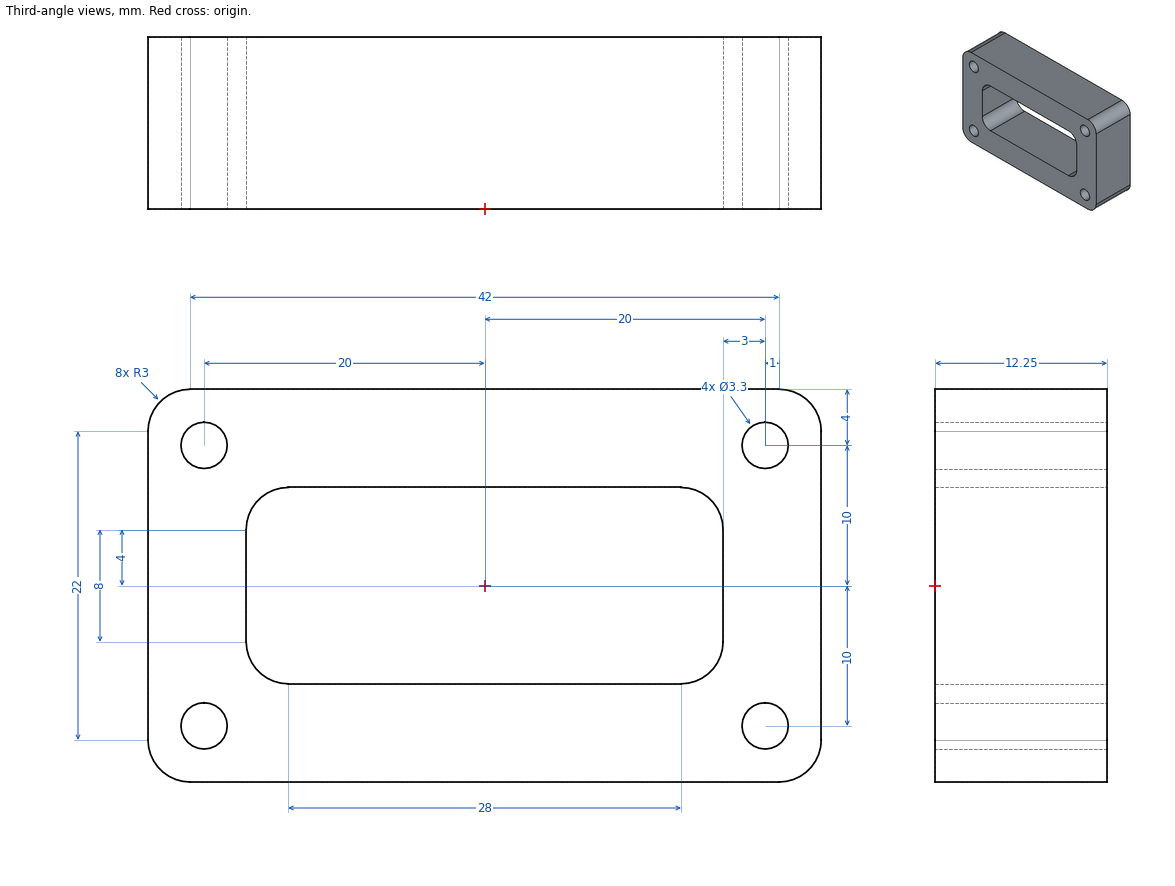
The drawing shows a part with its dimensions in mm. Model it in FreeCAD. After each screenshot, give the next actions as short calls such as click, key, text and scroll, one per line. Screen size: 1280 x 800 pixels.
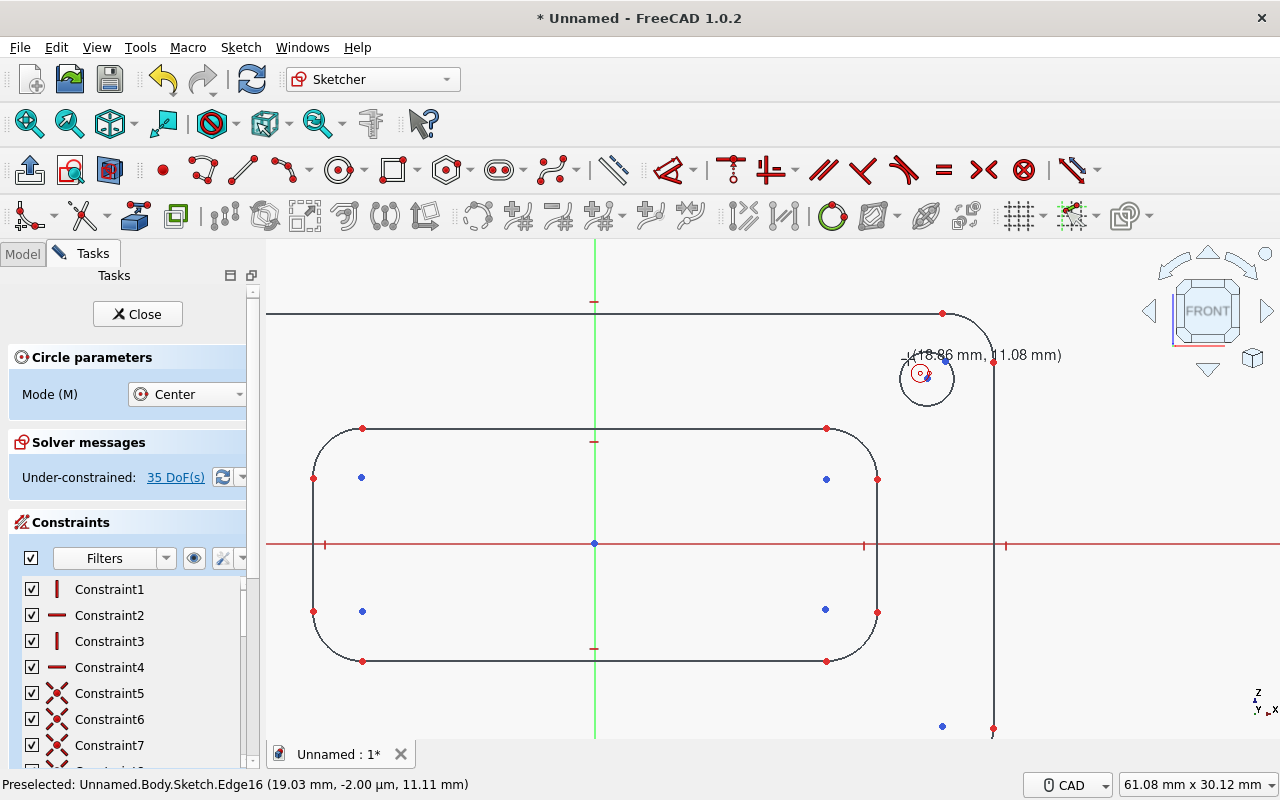
scroll(927, 377, down, 2)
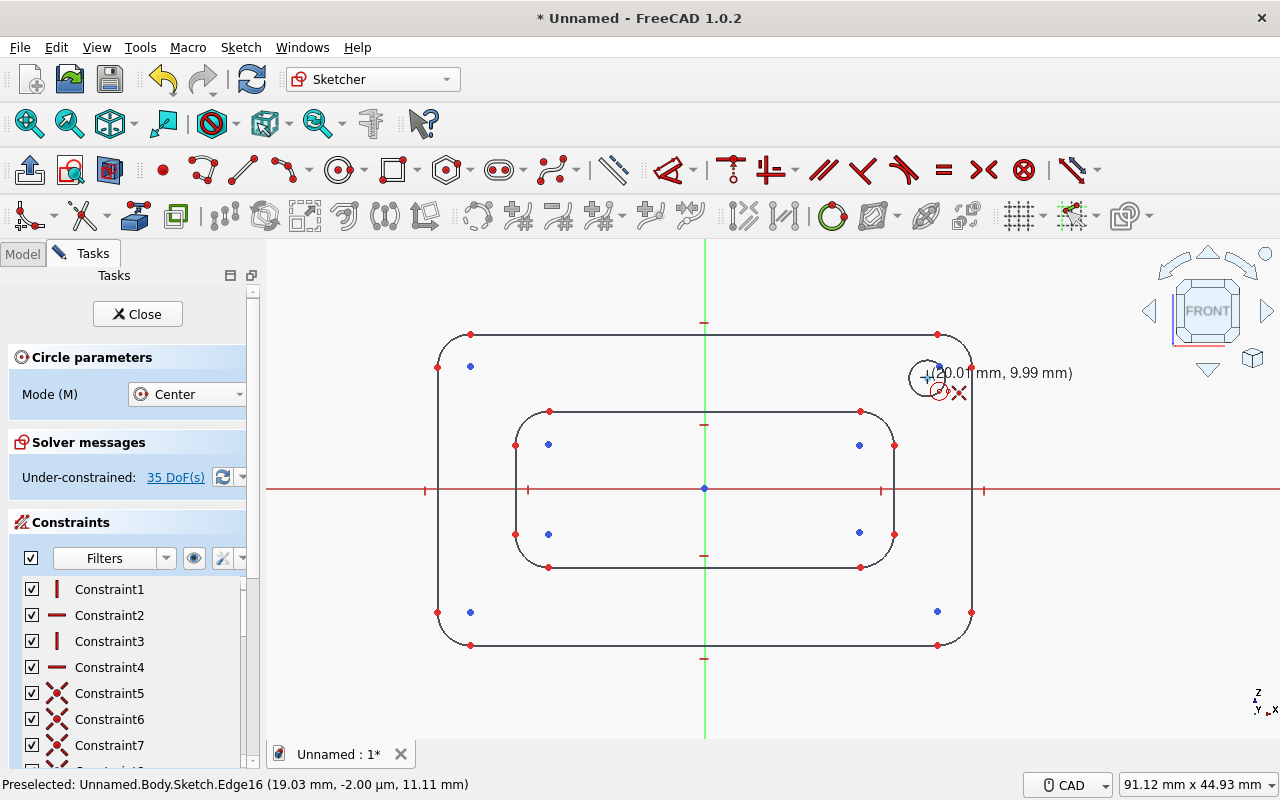
scroll(482, 378, up, 2)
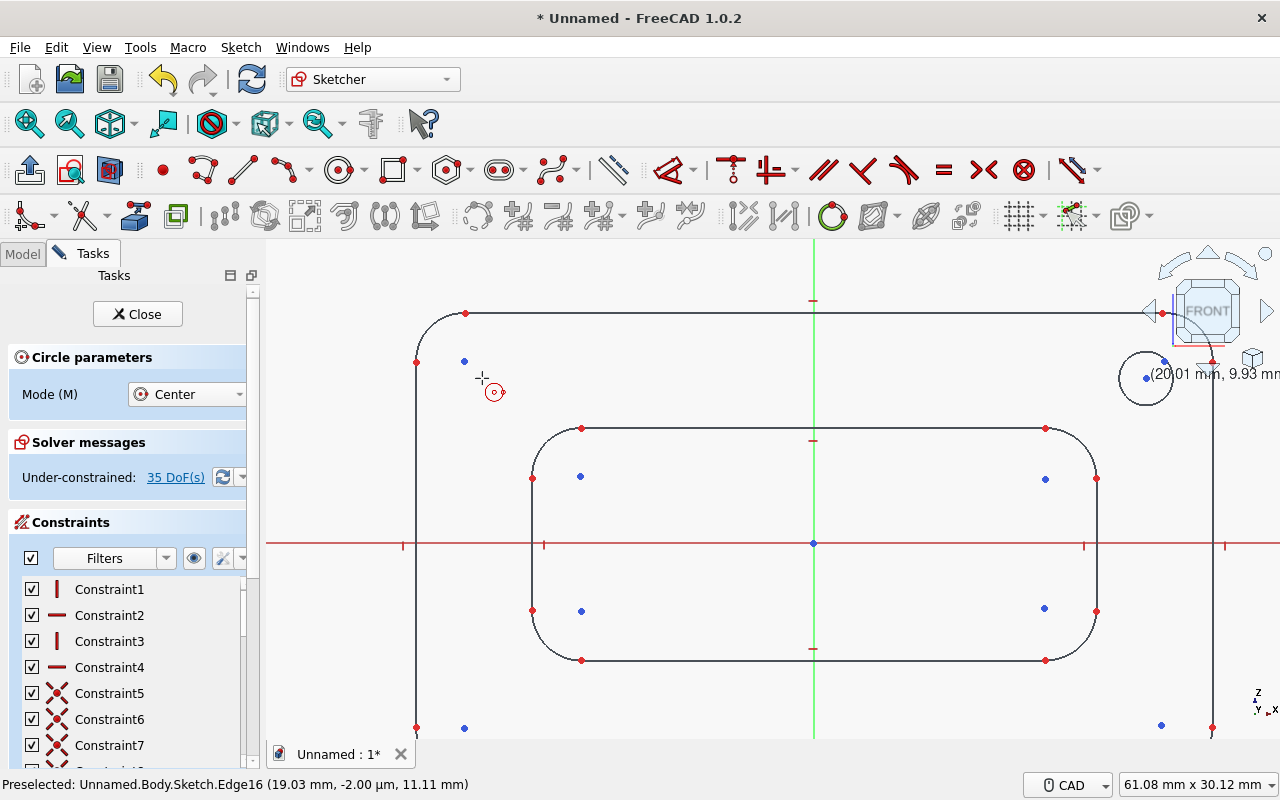
click(482, 377)
click(501, 358)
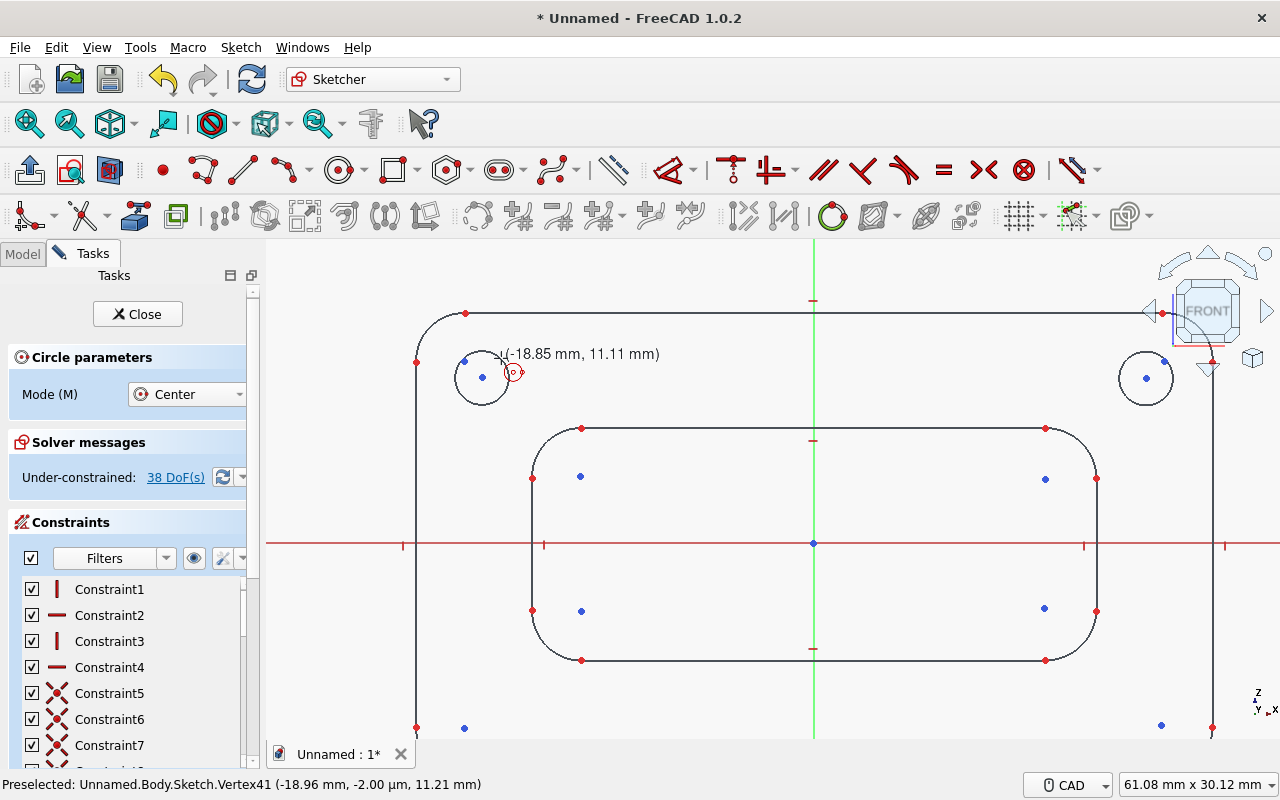
scroll(482, 378, down, 2)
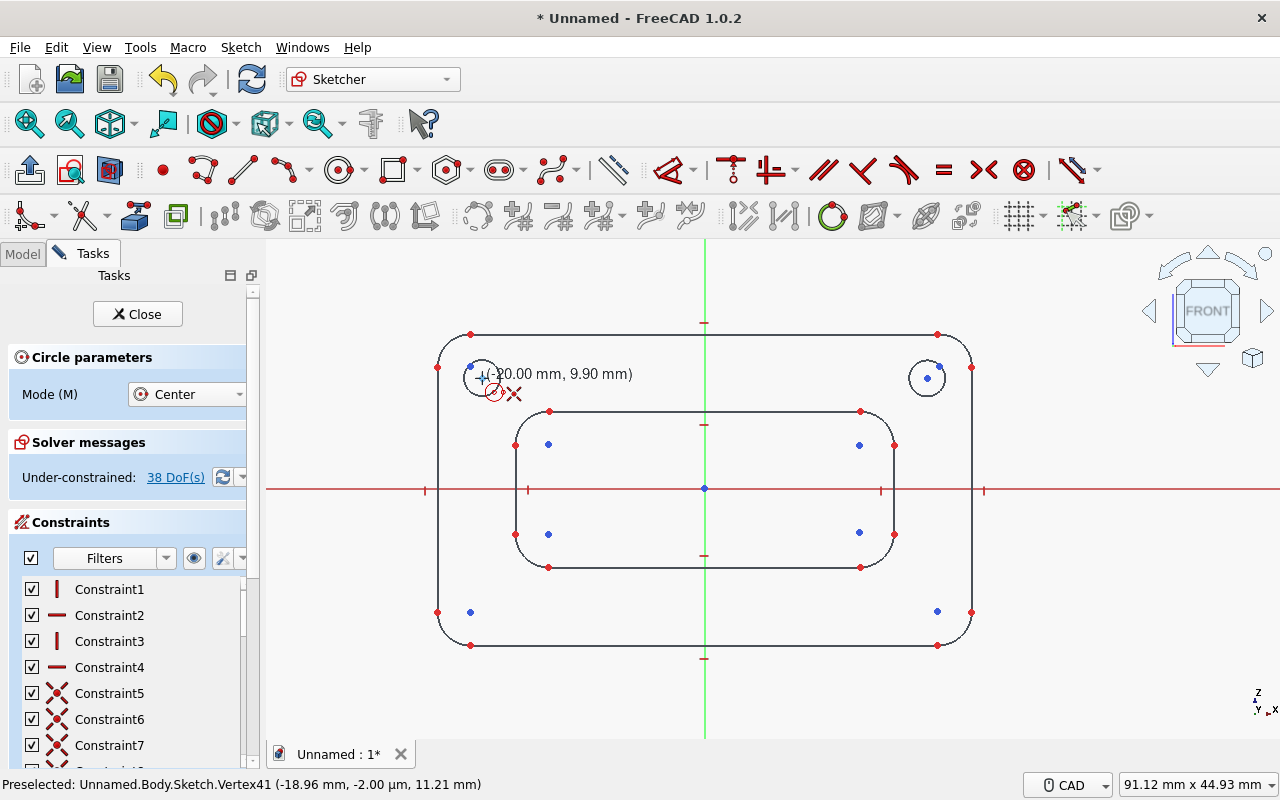
scroll(927, 600, up, 2)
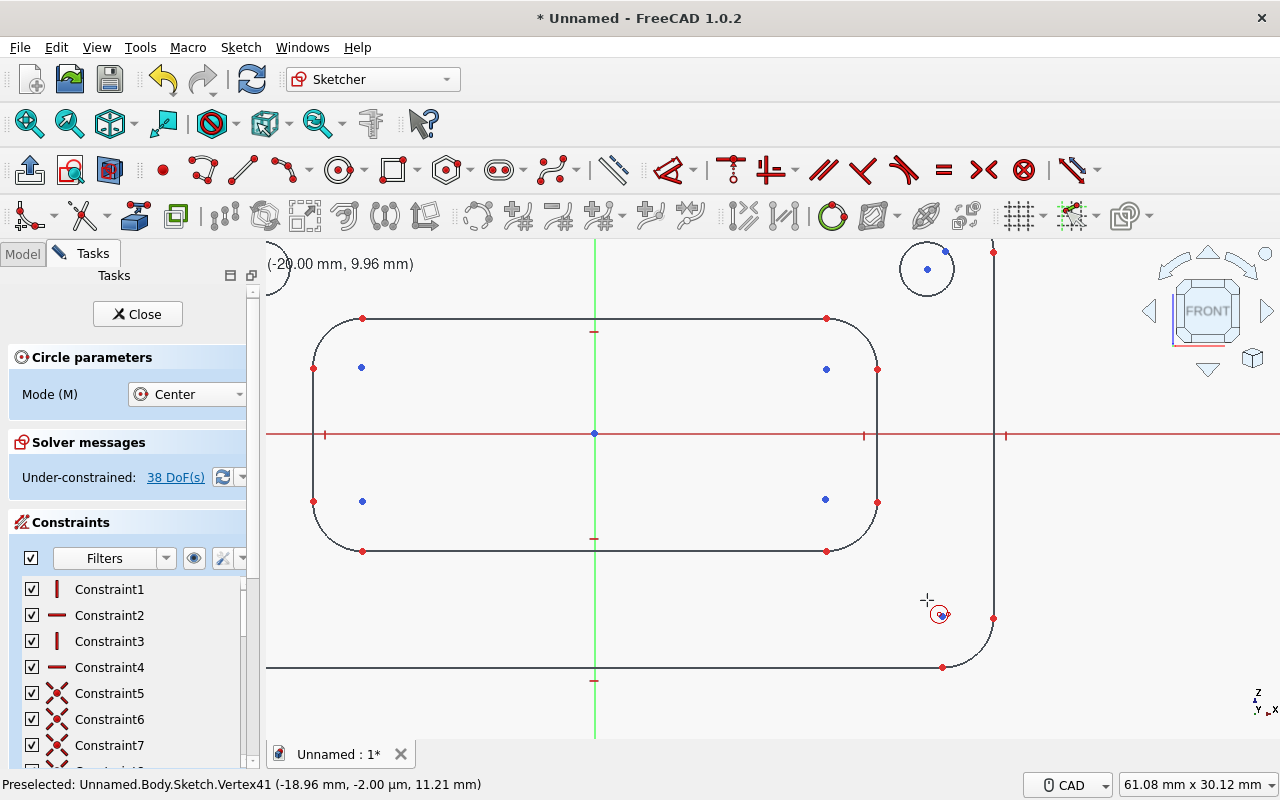
click(927, 600)
click(946, 581)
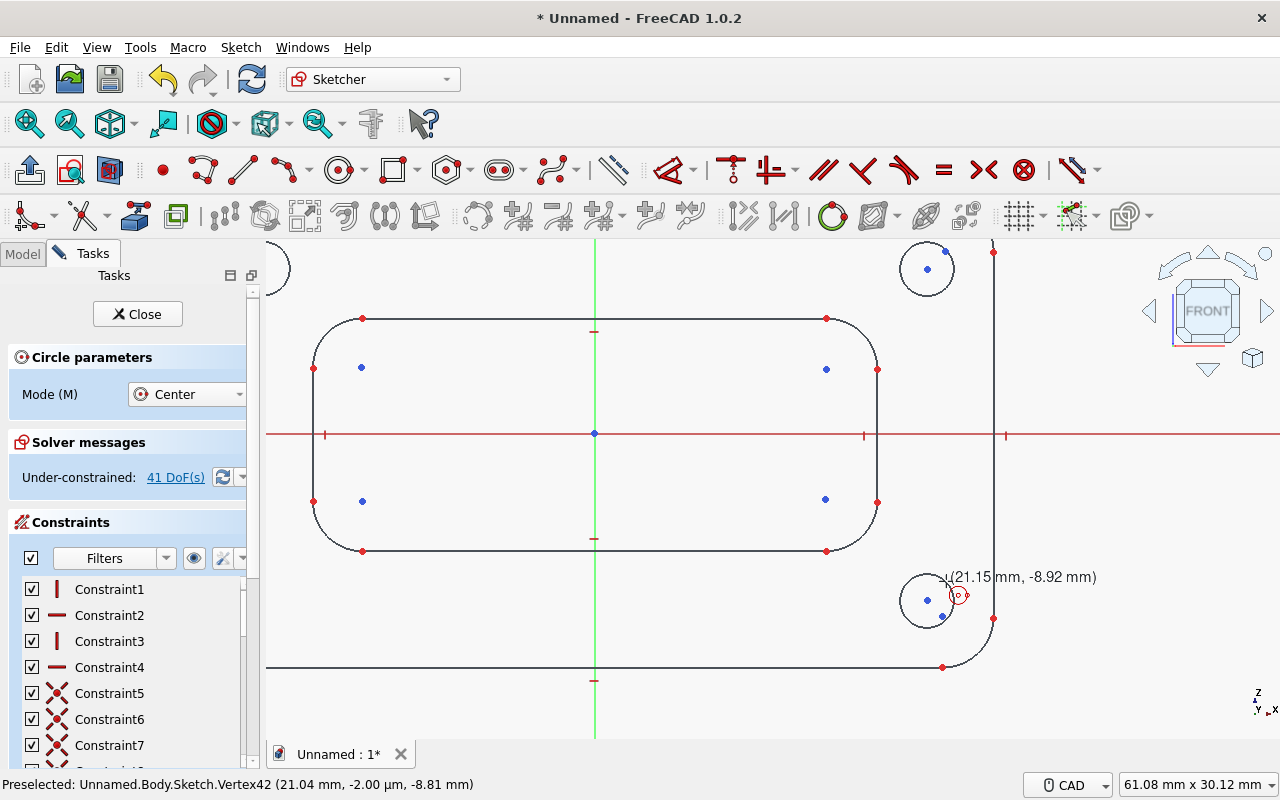
scroll(927, 601, down, 2)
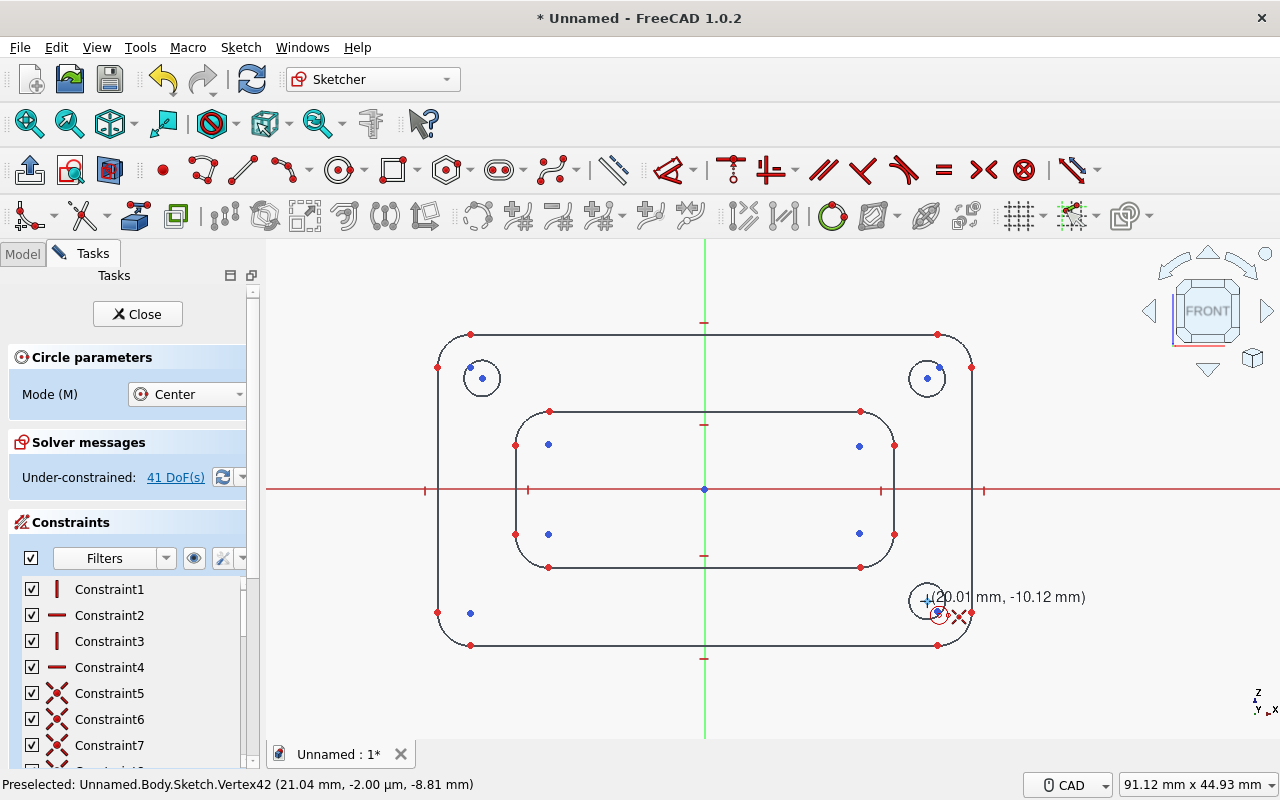
scroll(482, 601, up, 2)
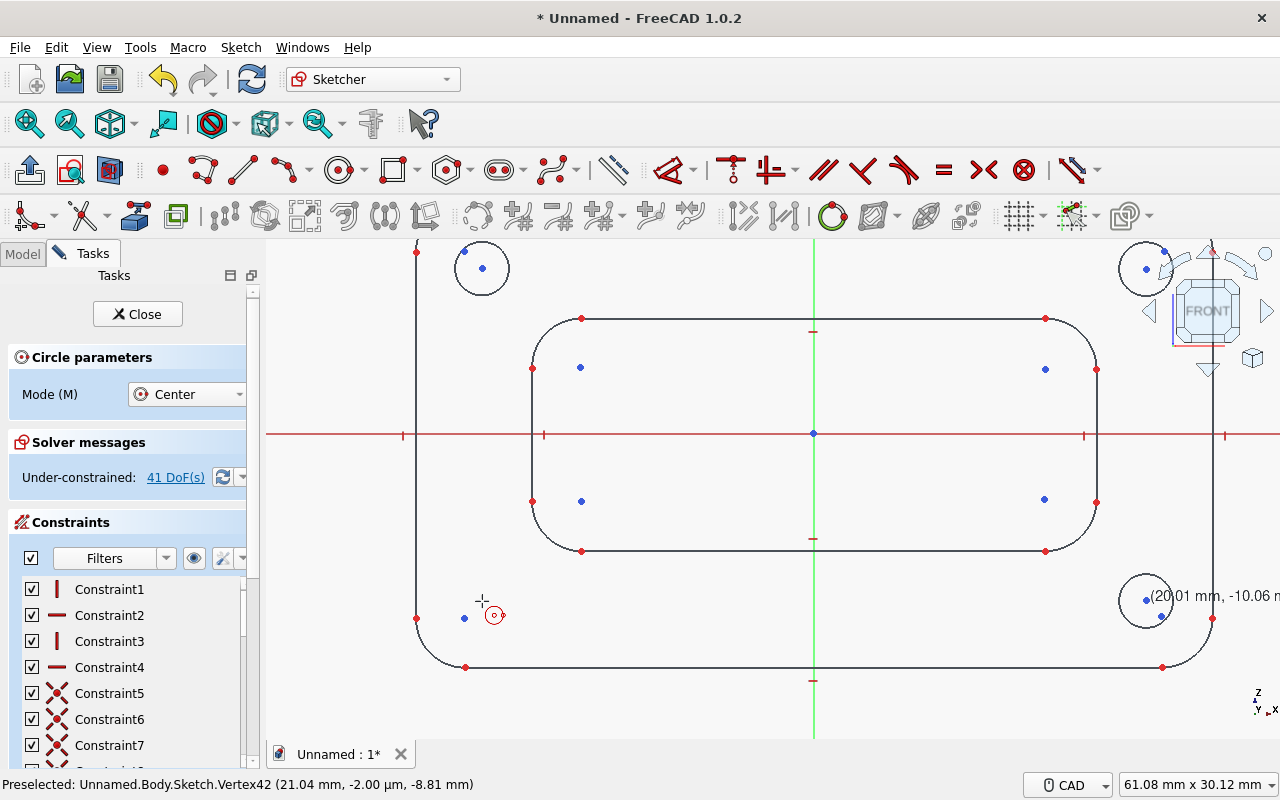
click(482, 600)
click(501, 581)
key(Escape)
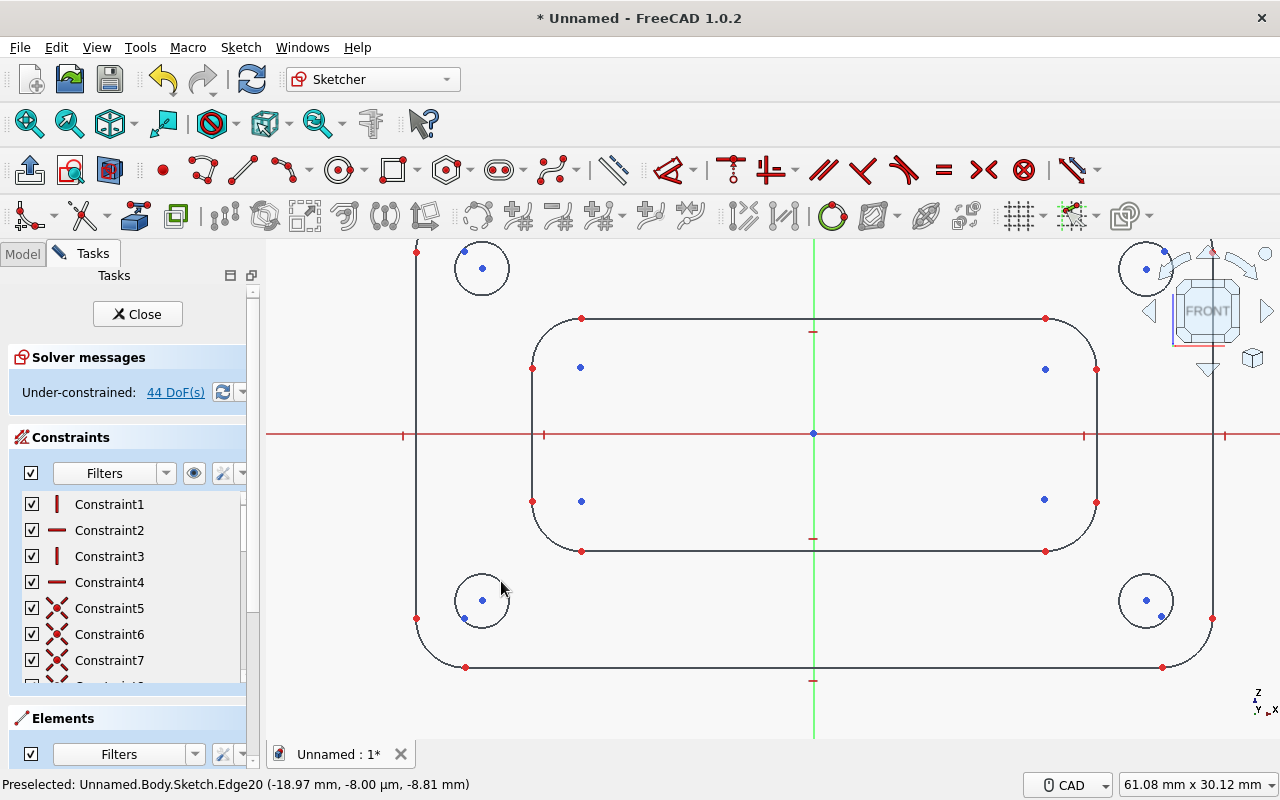
click(416, 509)